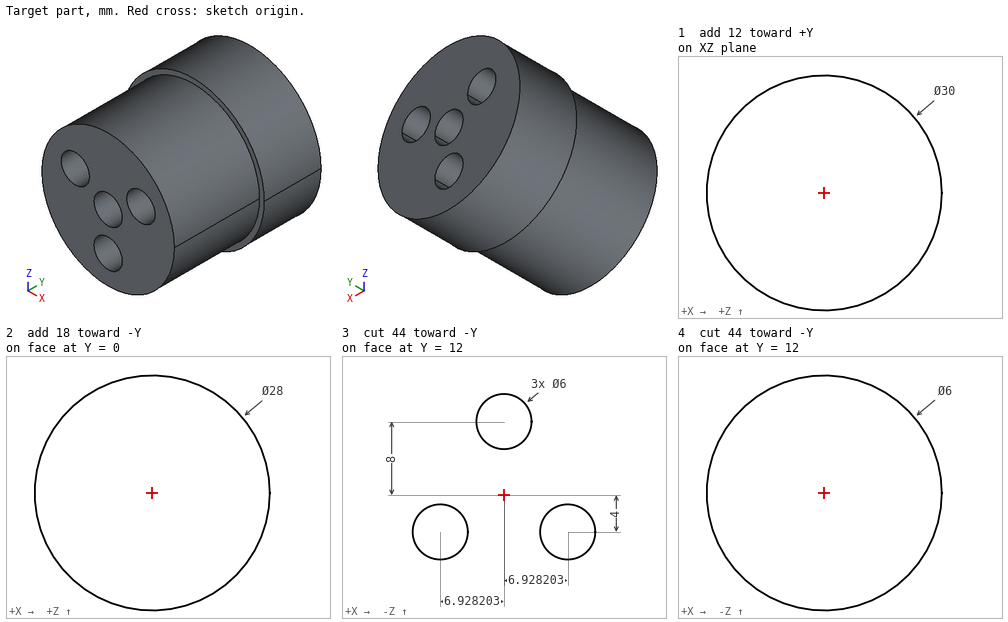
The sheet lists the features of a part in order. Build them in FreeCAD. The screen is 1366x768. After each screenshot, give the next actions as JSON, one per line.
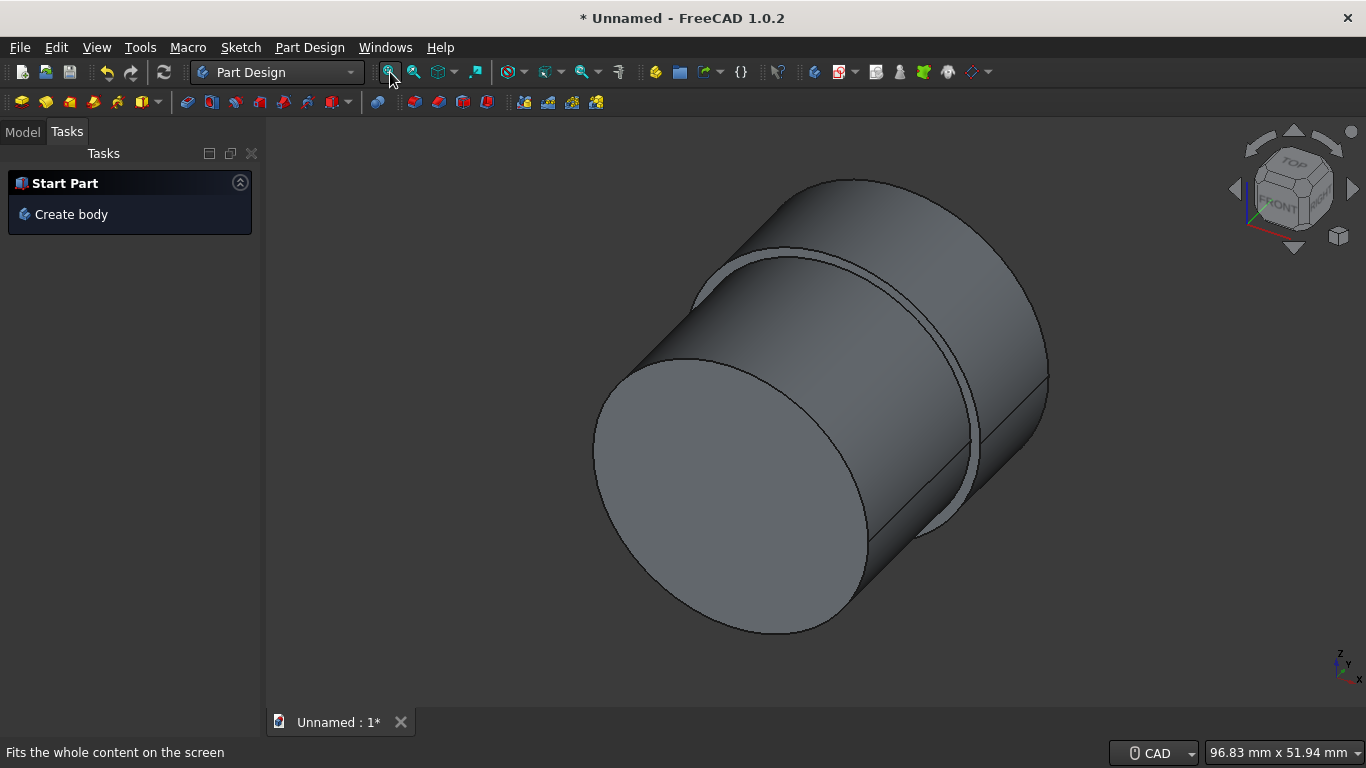
{"action": "key", "text": "4"}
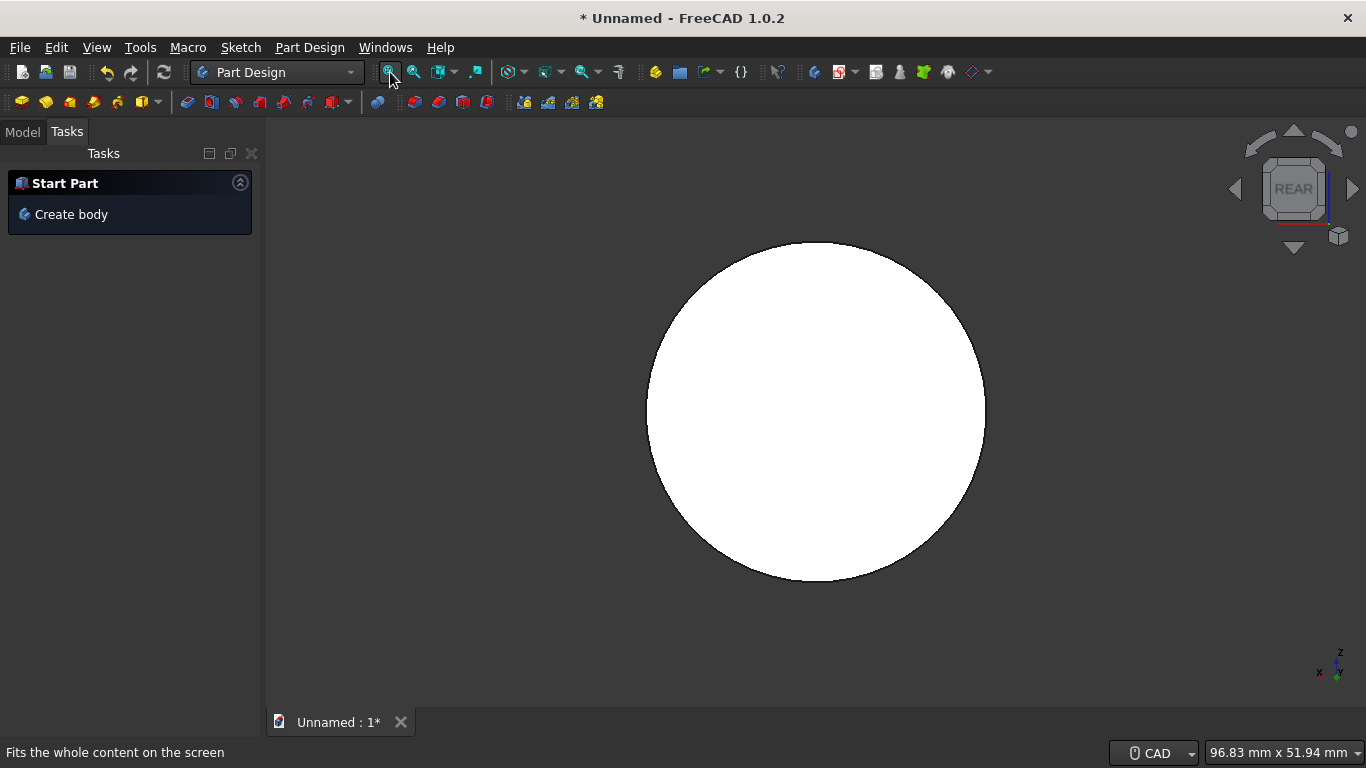
{"action": "left_click", "coordinate": [816, 411]}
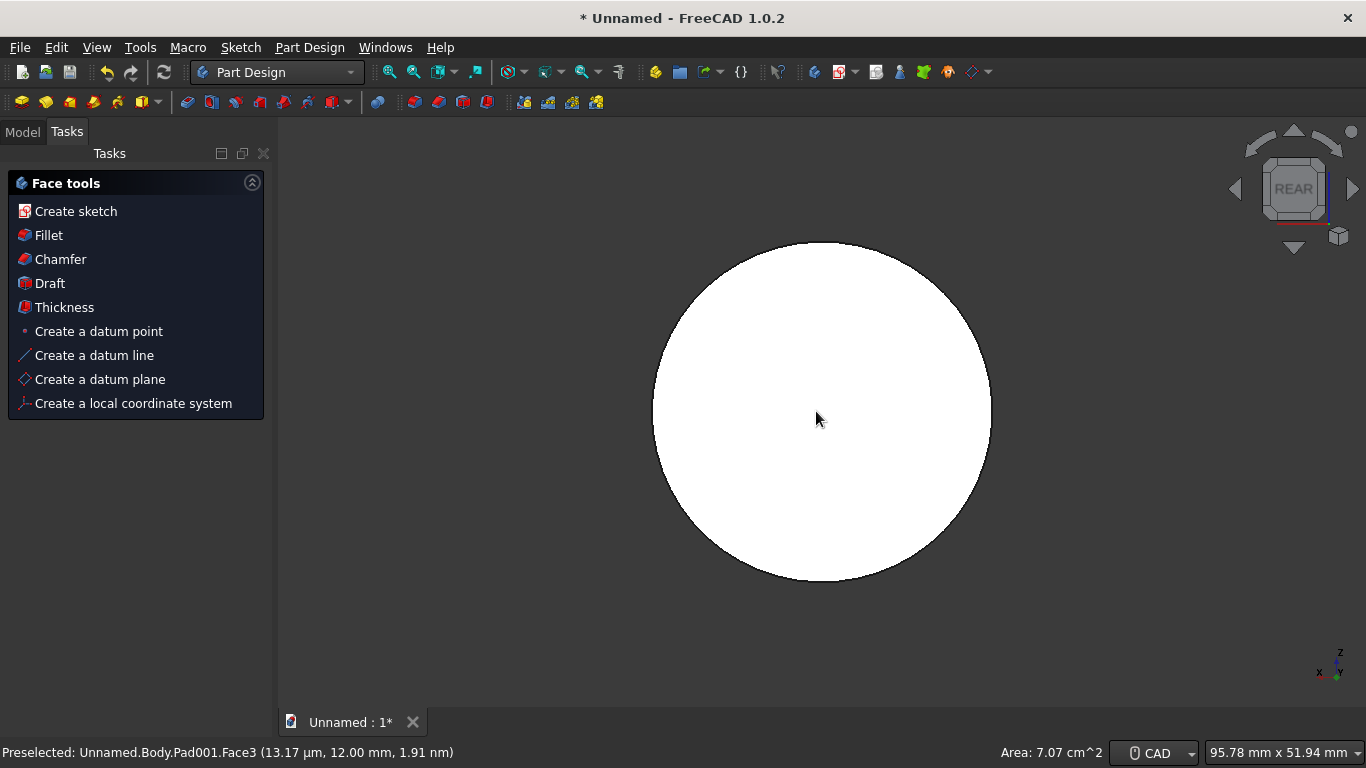
{"action": "left_click", "coordinate": [840, 72]}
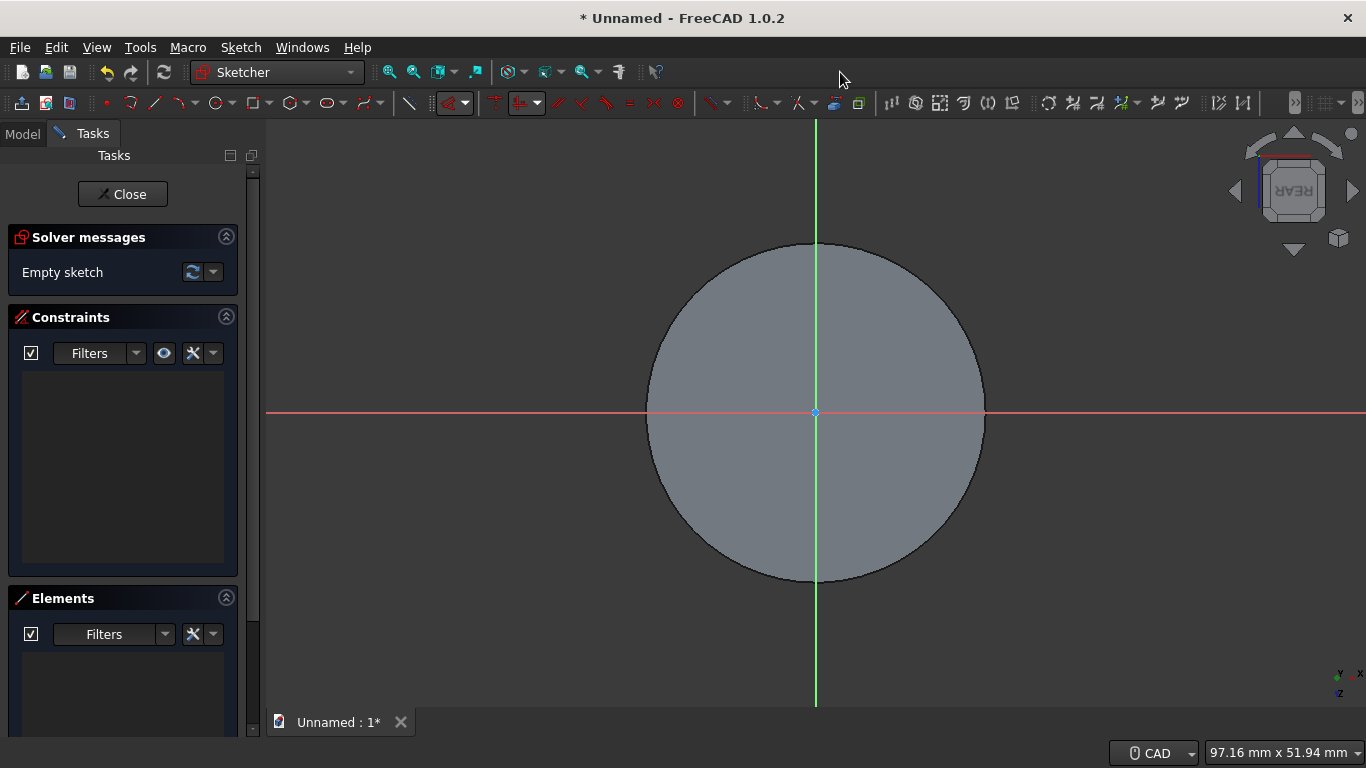
{"action": "scroll", "coordinate": [899, 363], "scroll_direction": "up", "scroll_amount": 3}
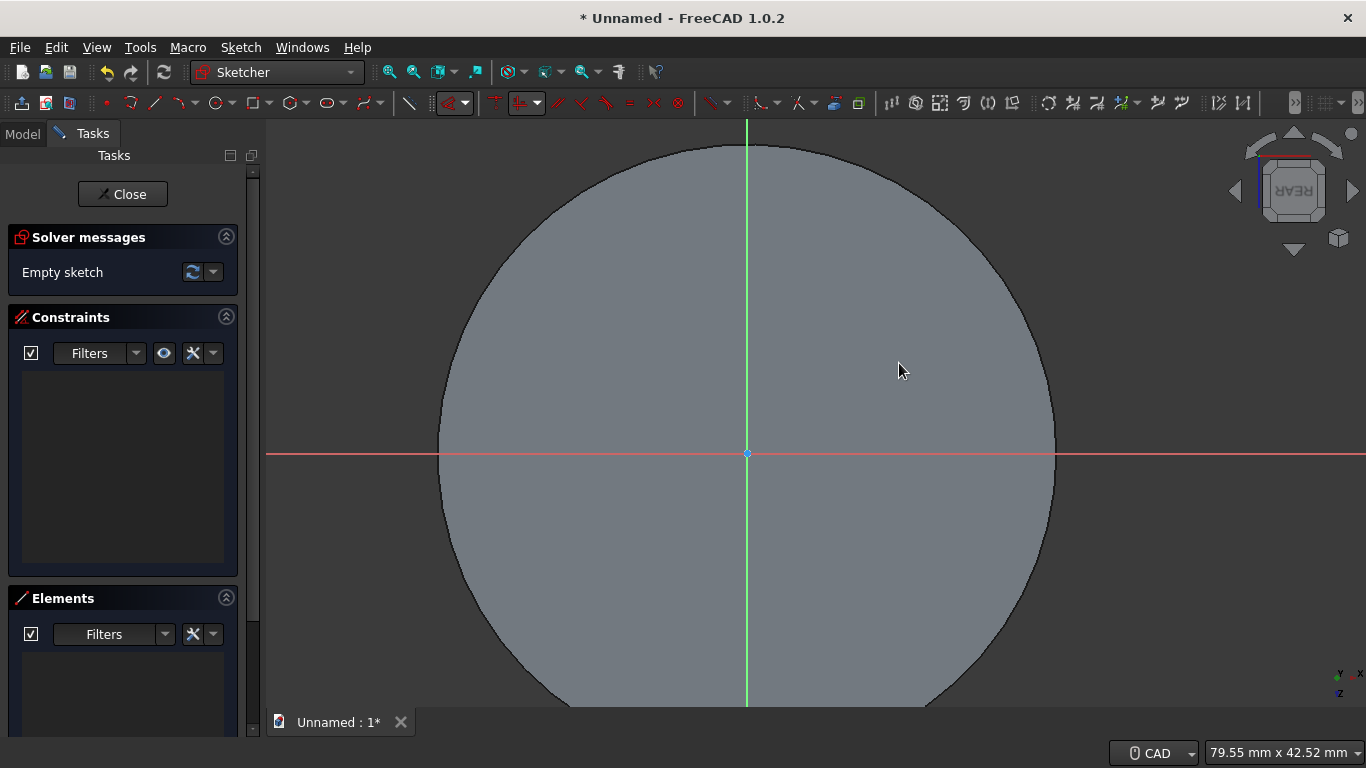
{"action": "left_click", "coordinate": [216, 104]}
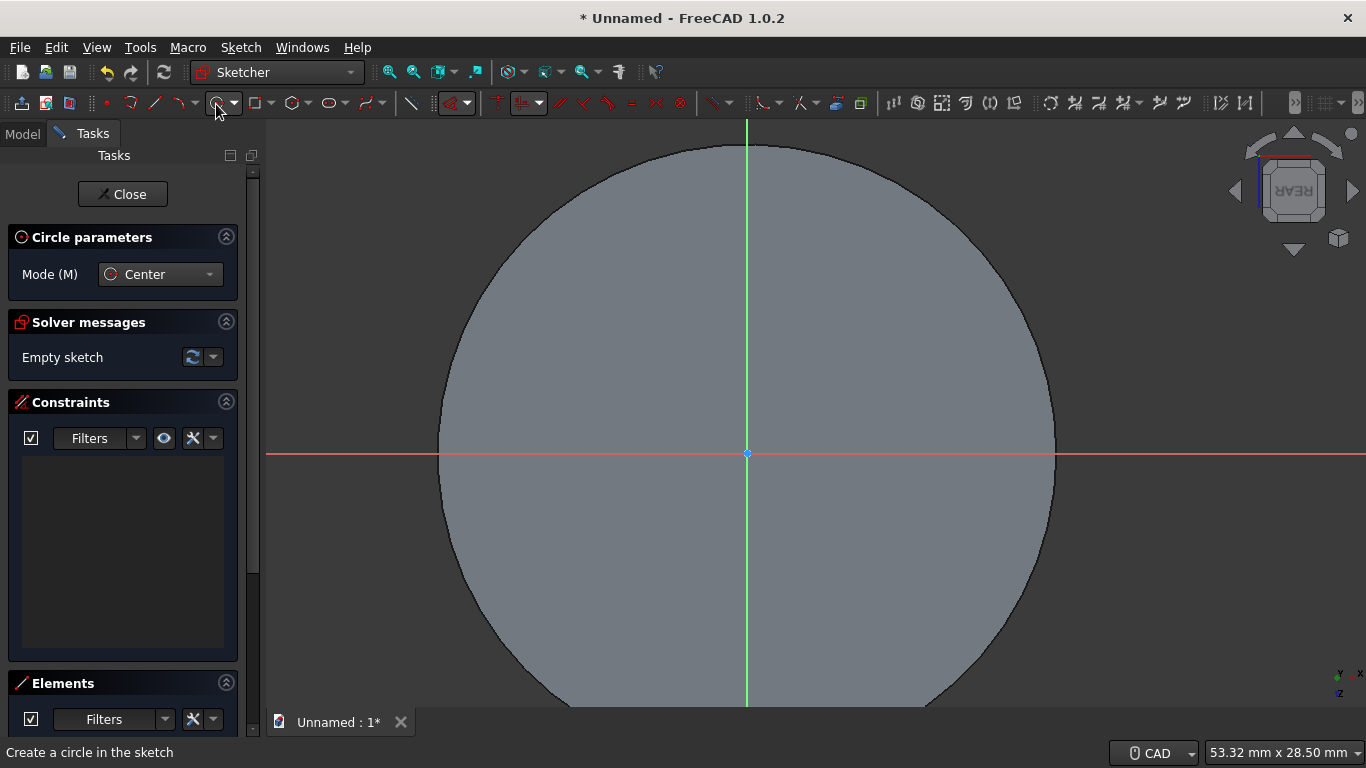
{"action": "left_click", "coordinate": [747, 289]}
{"action": "left_click", "coordinate": [791, 245]}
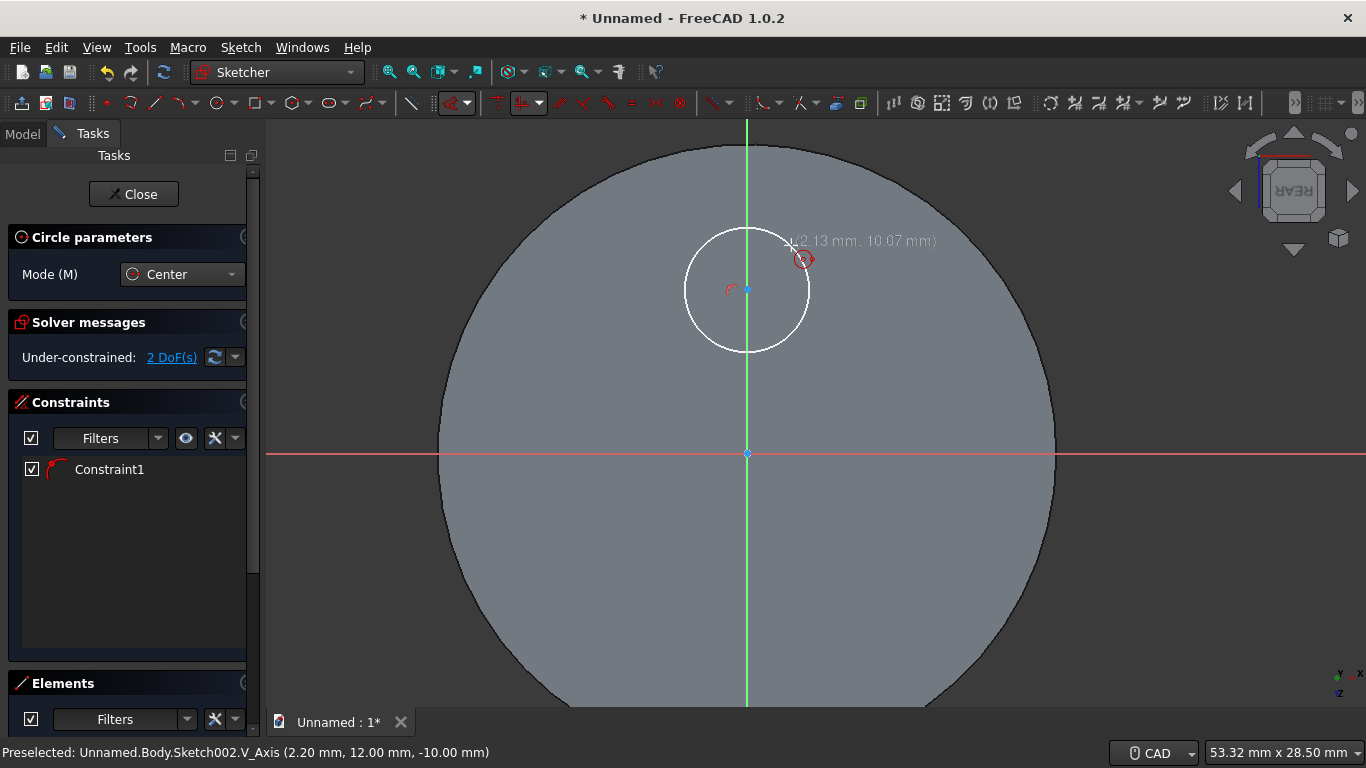
{"action": "left_click", "coordinate": [890, 536]}
{"action": "left_click", "coordinate": [934, 493]}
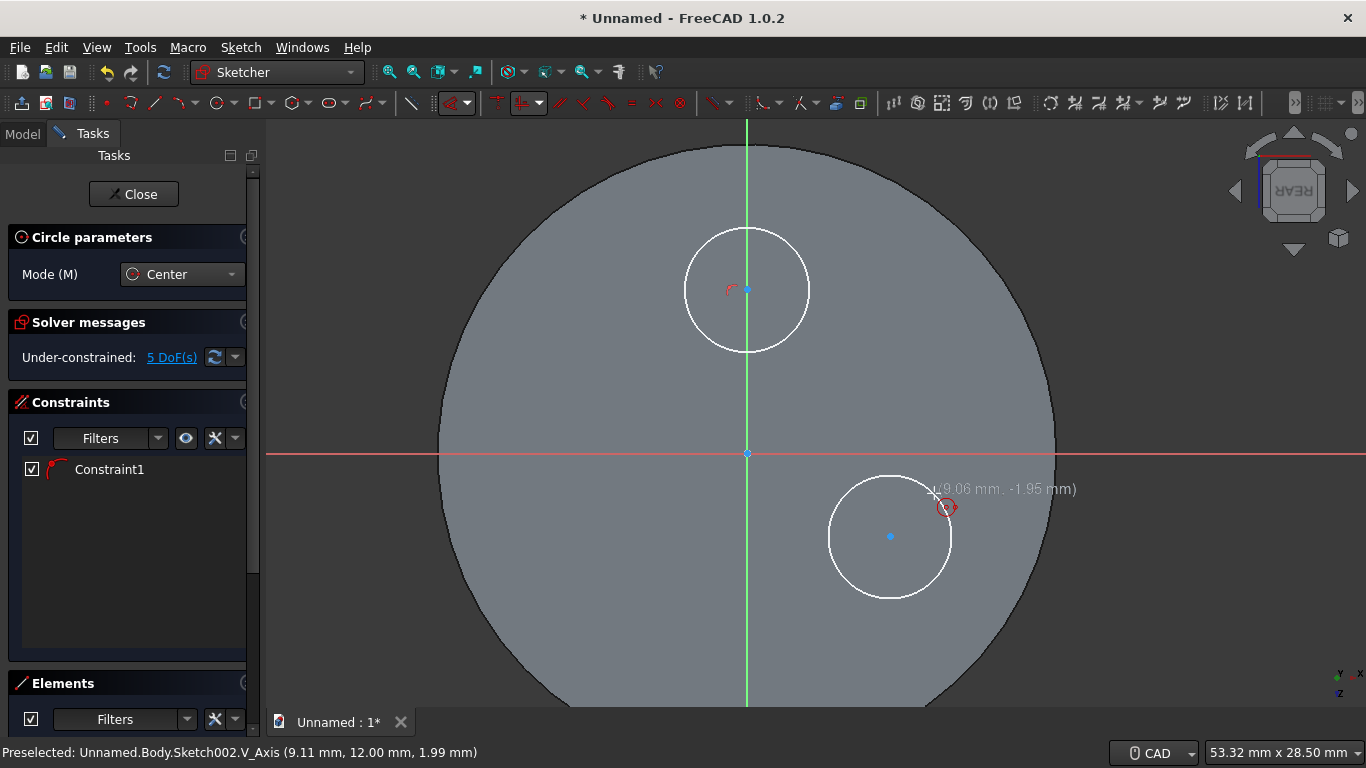
{"action": "left_click", "coordinate": [604, 536]}
{"action": "left_click", "coordinate": [648, 493]}
{"action": "key", "text": "Escape"}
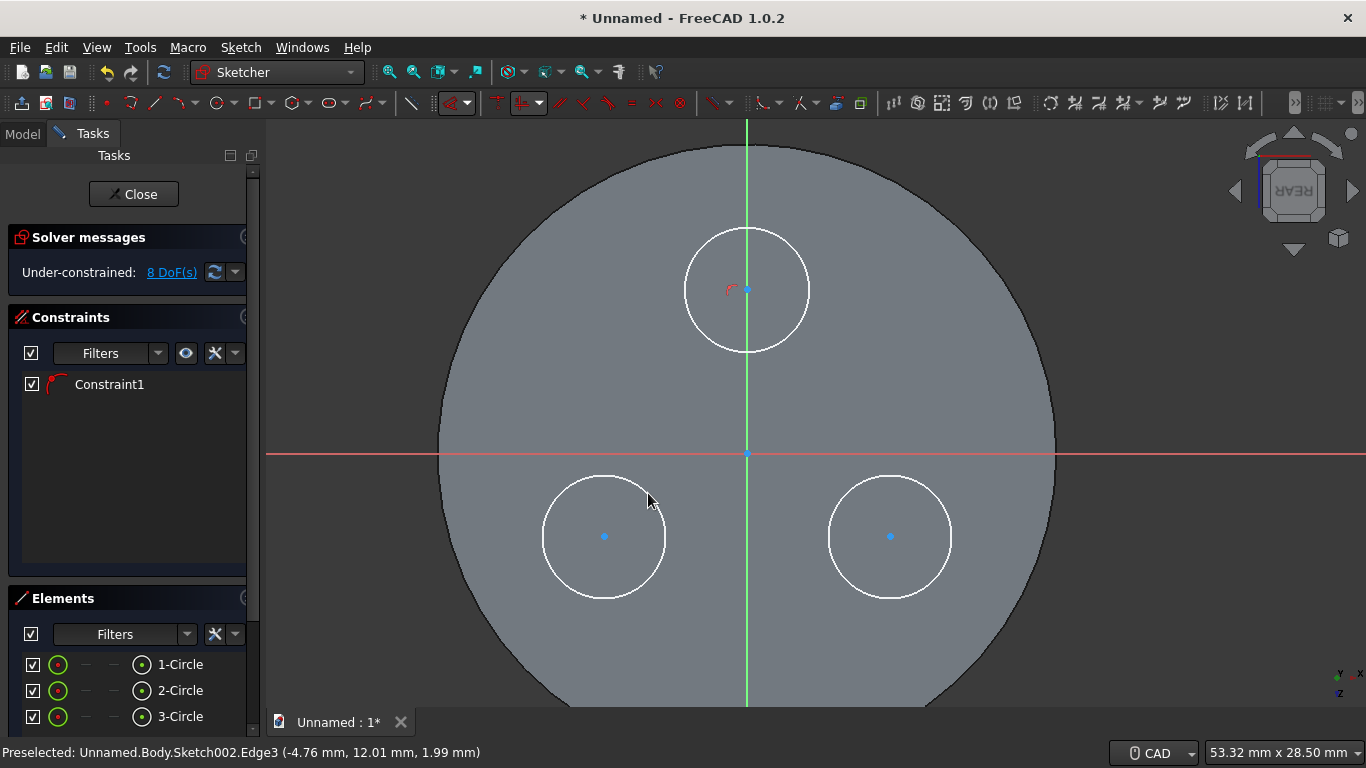
{"action": "left_click", "coordinate": [791, 246]}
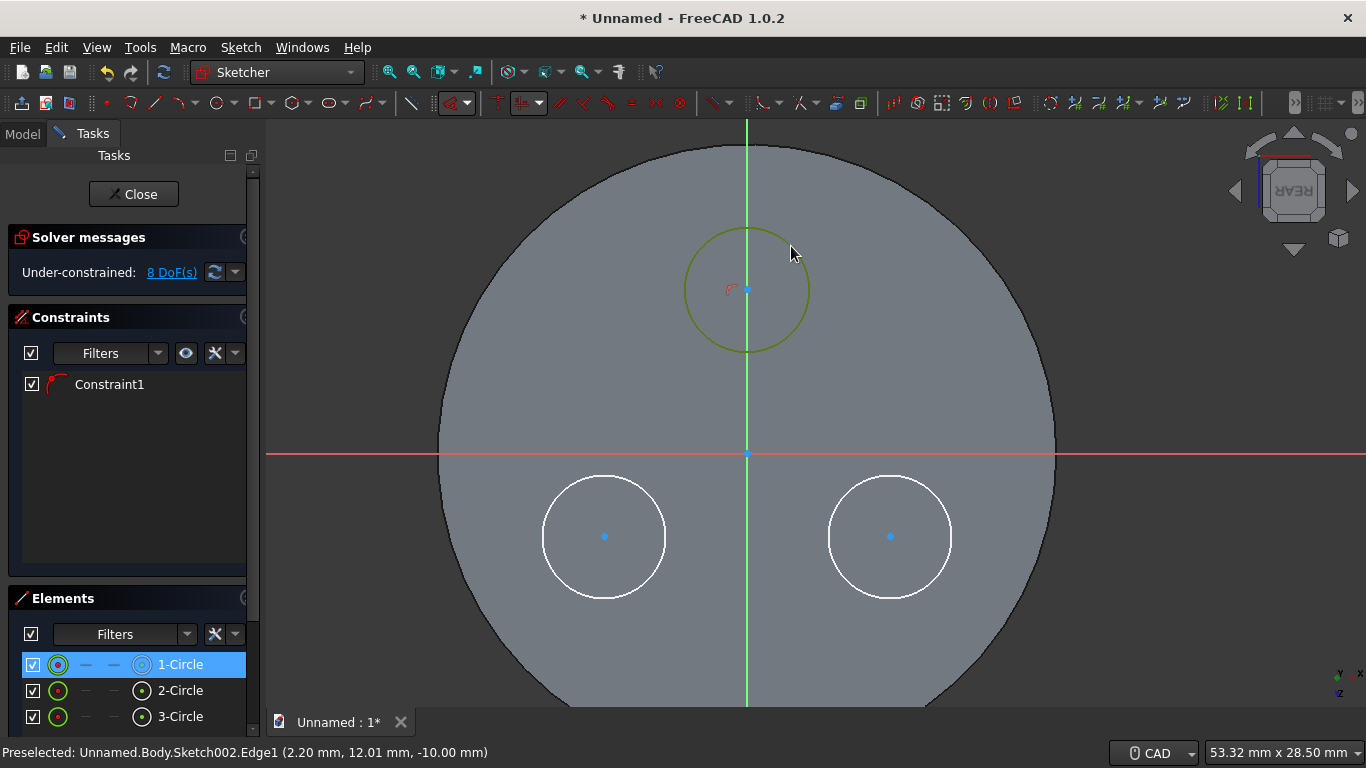
{"action": "left_click", "coordinate": [933, 493]}